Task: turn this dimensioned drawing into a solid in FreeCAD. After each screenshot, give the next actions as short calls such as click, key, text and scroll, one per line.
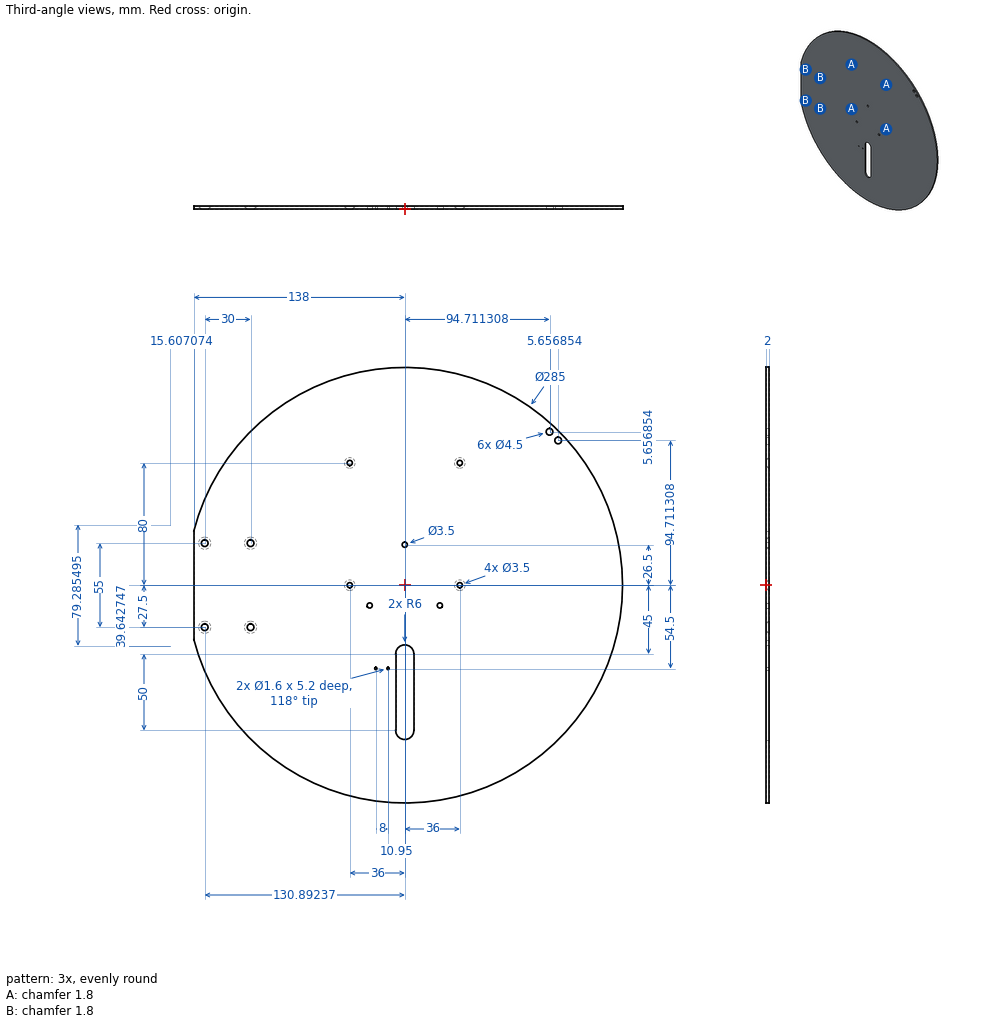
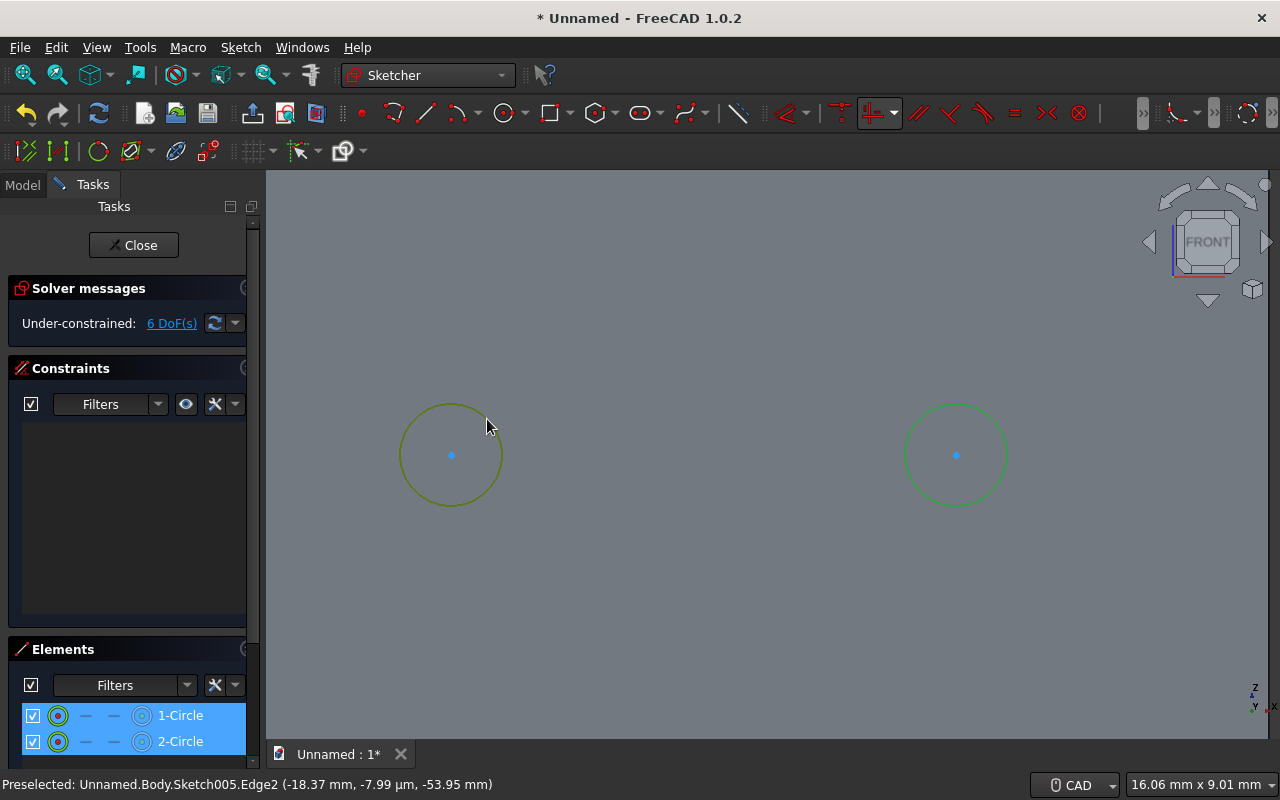
click(1016, 114)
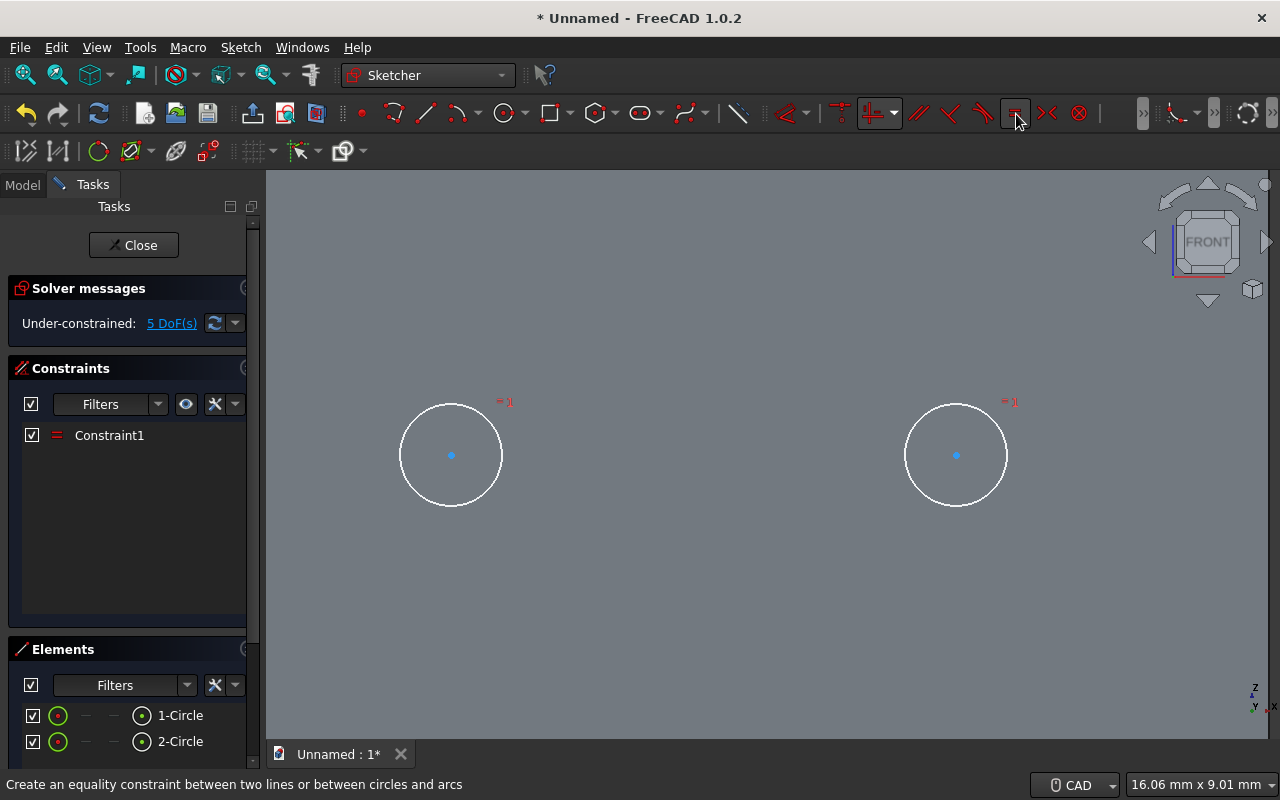
click(956, 455)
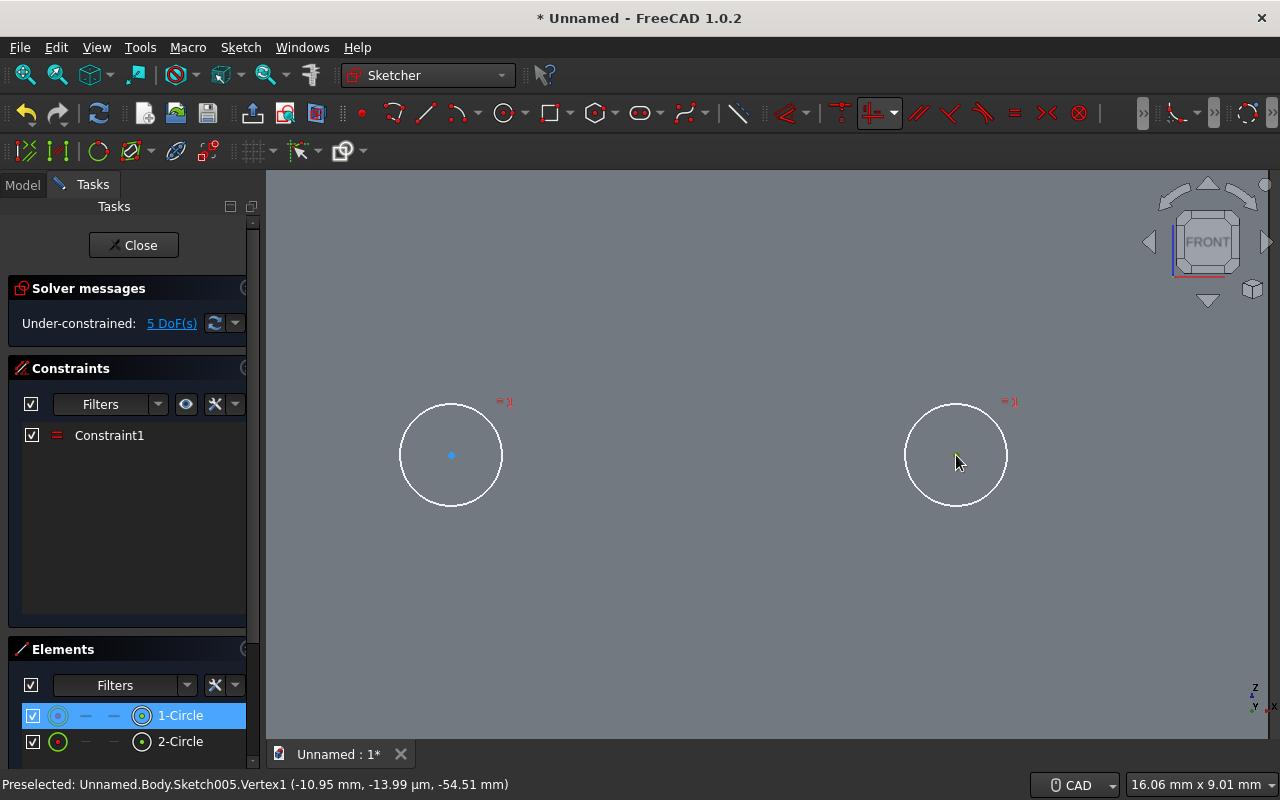
click(451, 455)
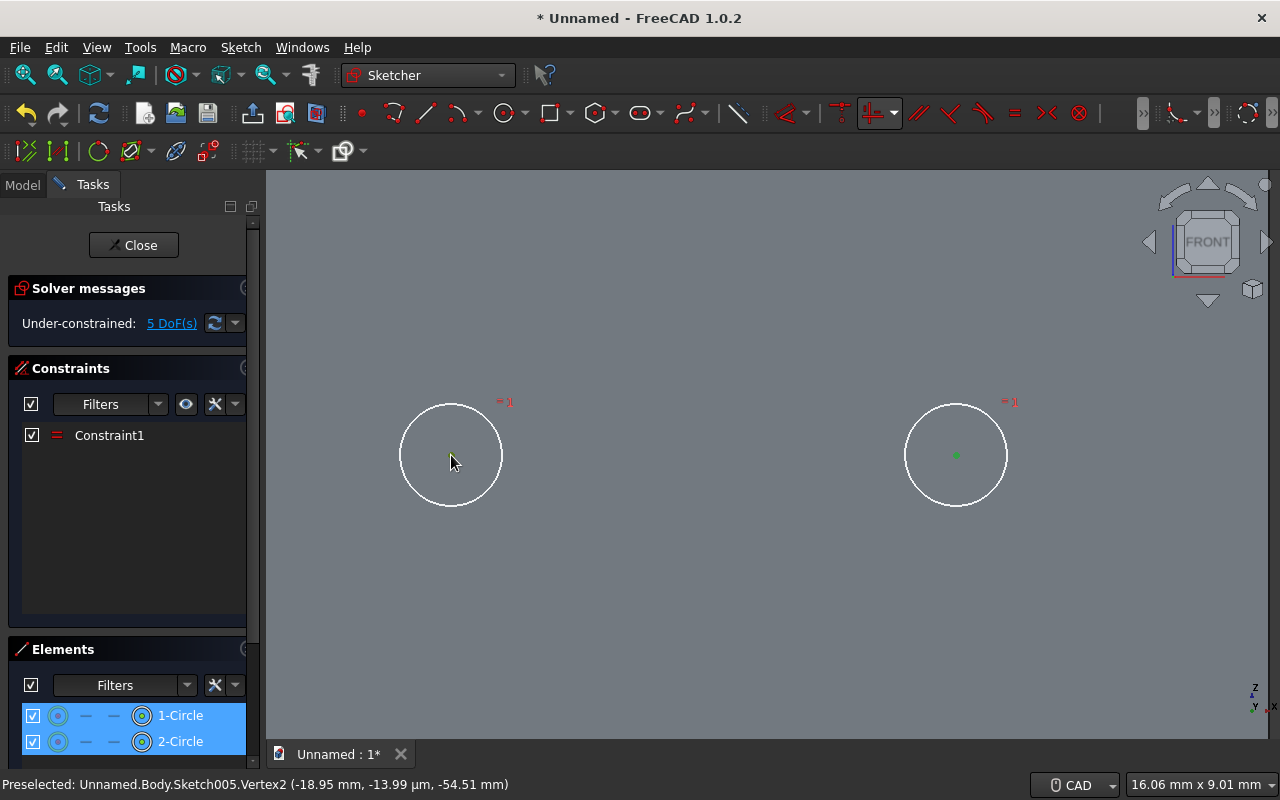
click(896, 114)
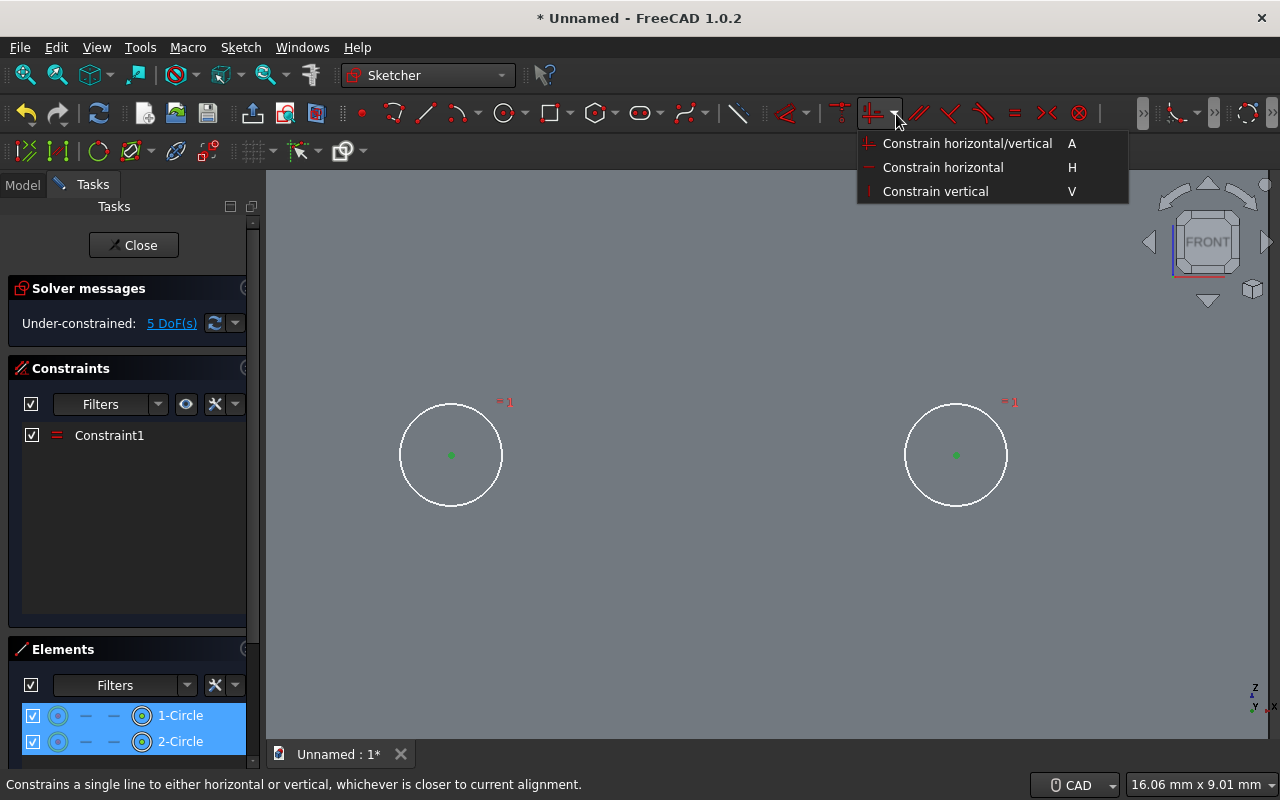
click(993, 167)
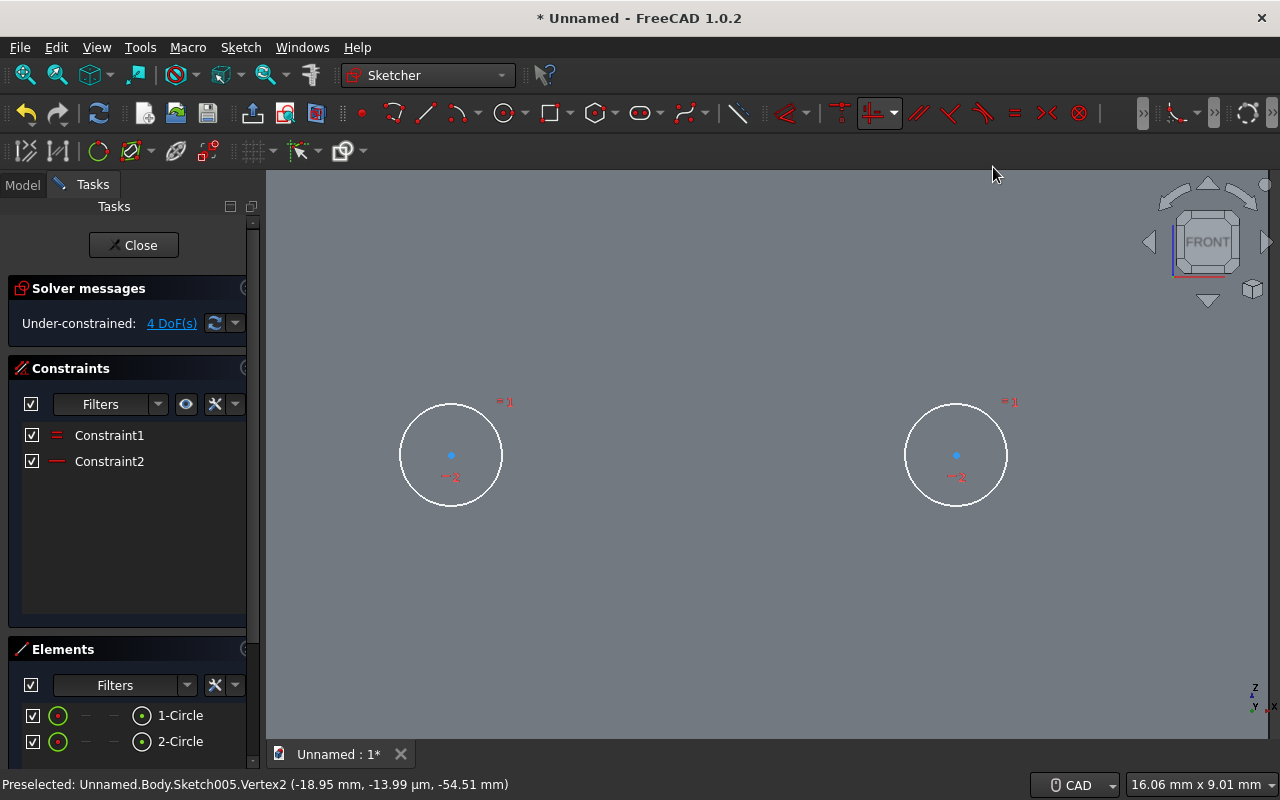
click(786, 114)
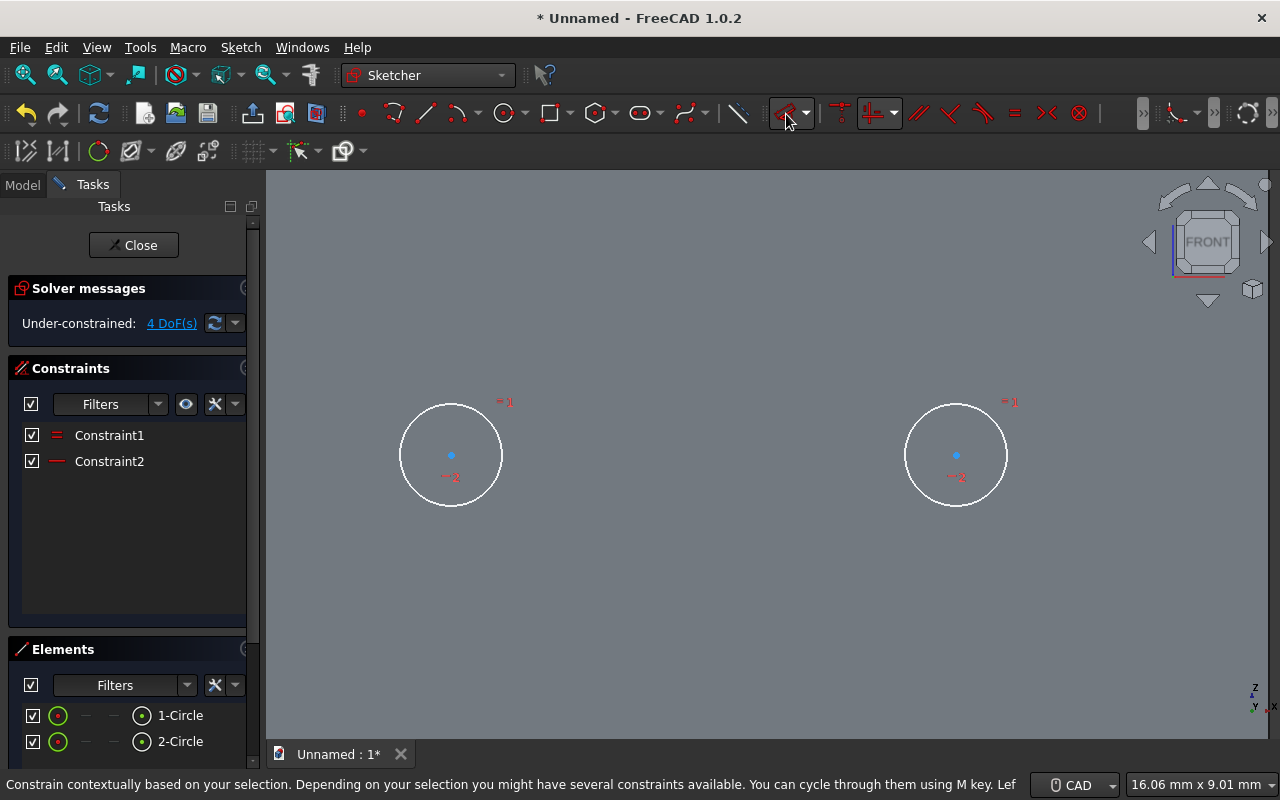
click(992, 419)
click(1015, 396)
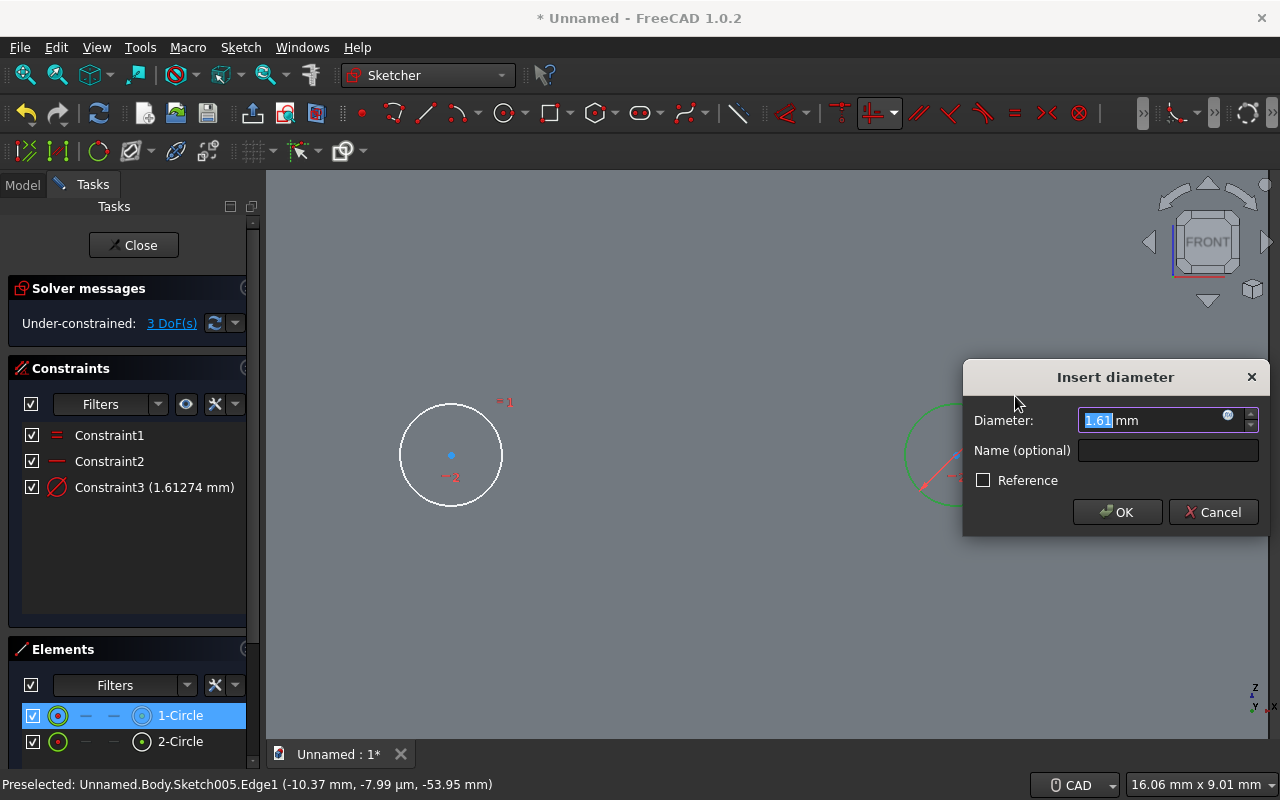
text(1.6)
key(Return)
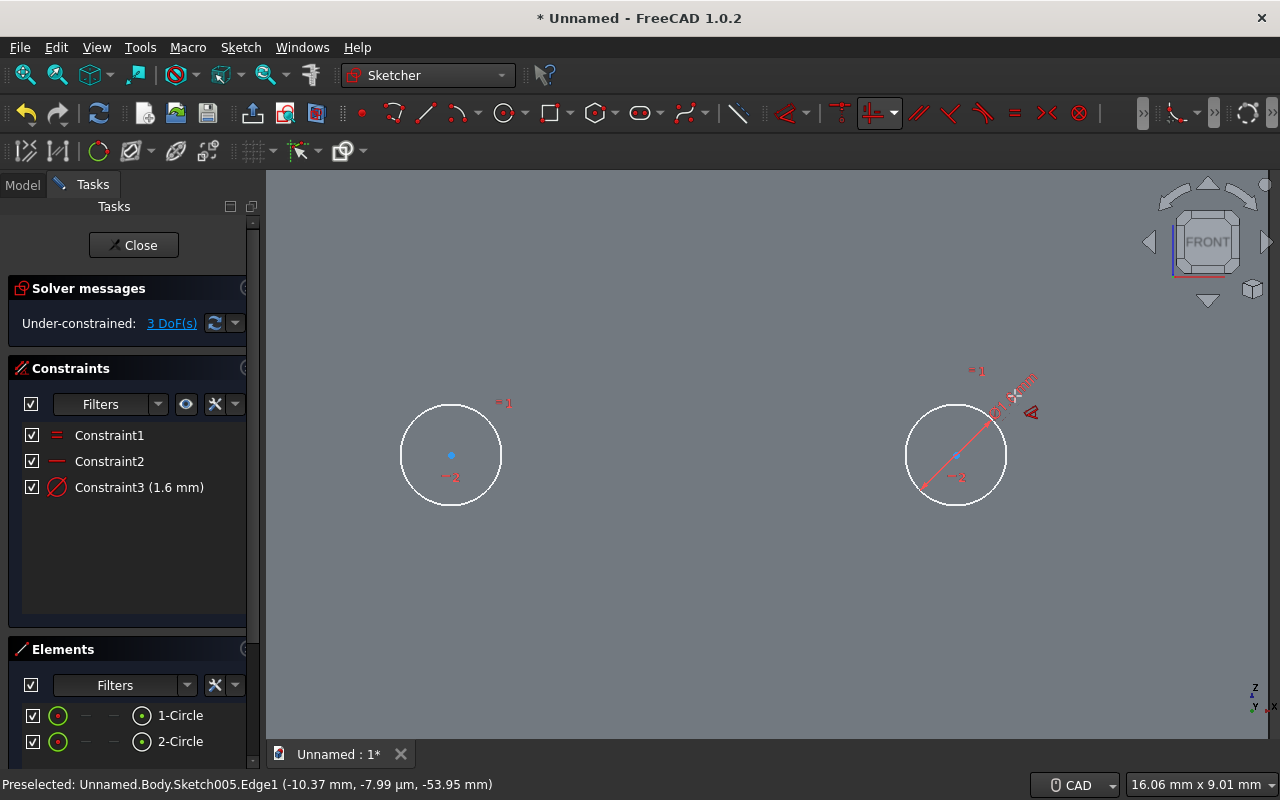
click(956, 455)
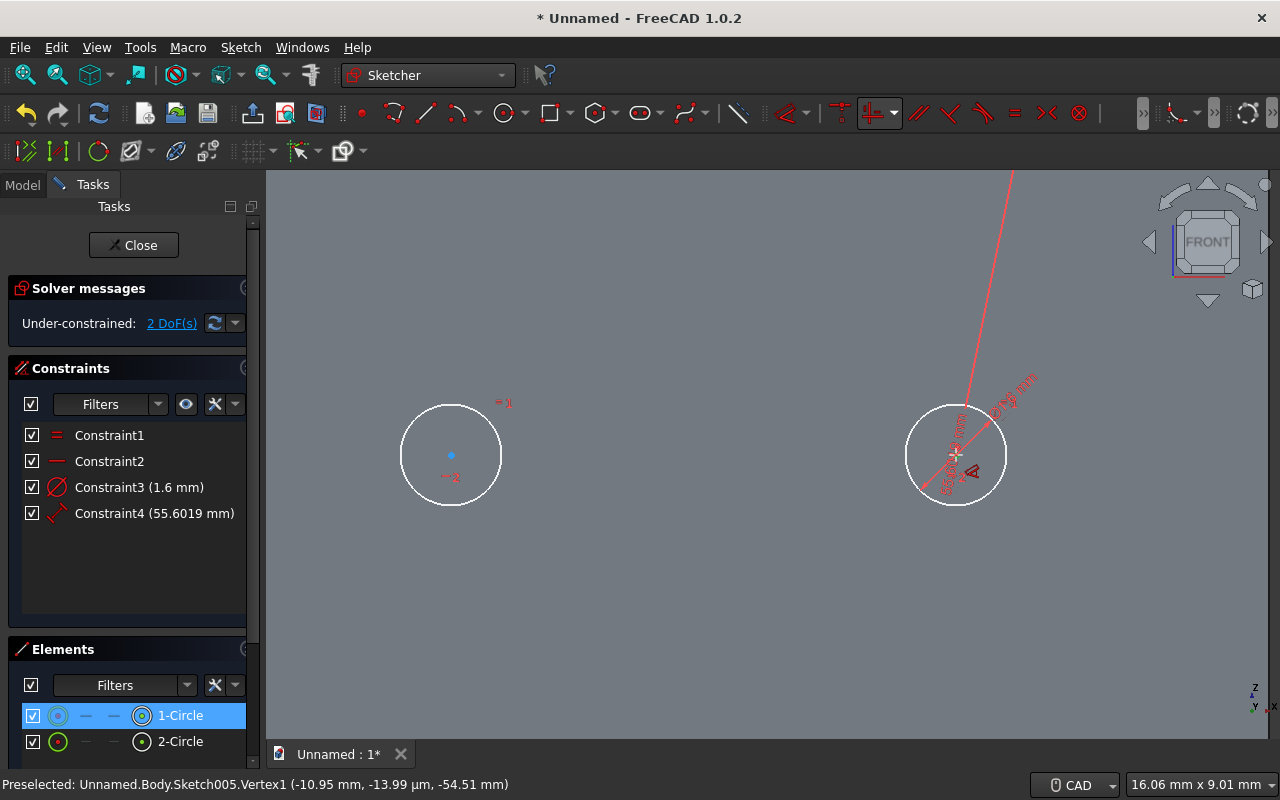
click(451, 455)
click(704, 489)